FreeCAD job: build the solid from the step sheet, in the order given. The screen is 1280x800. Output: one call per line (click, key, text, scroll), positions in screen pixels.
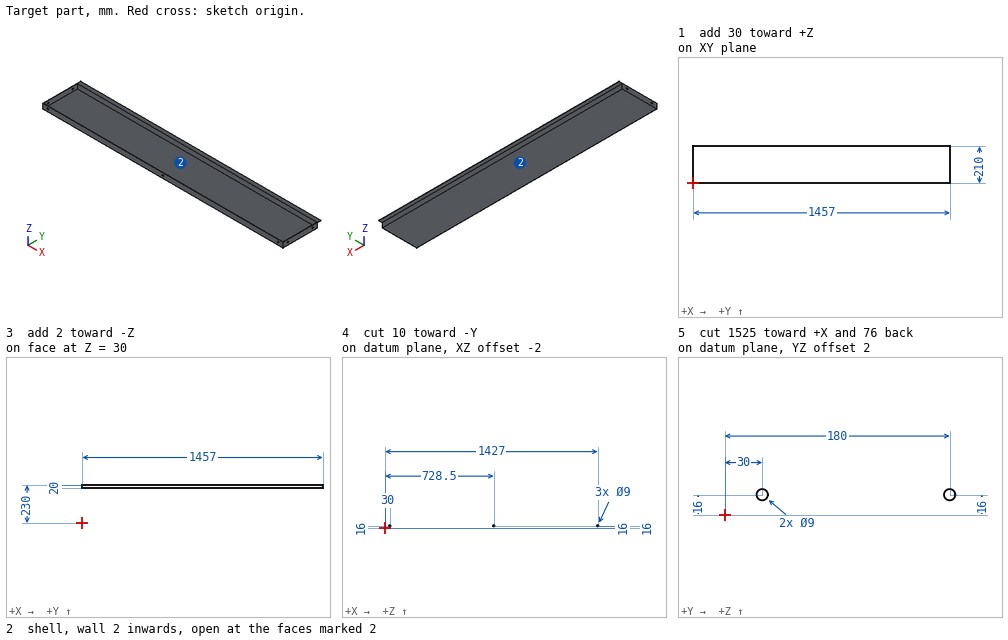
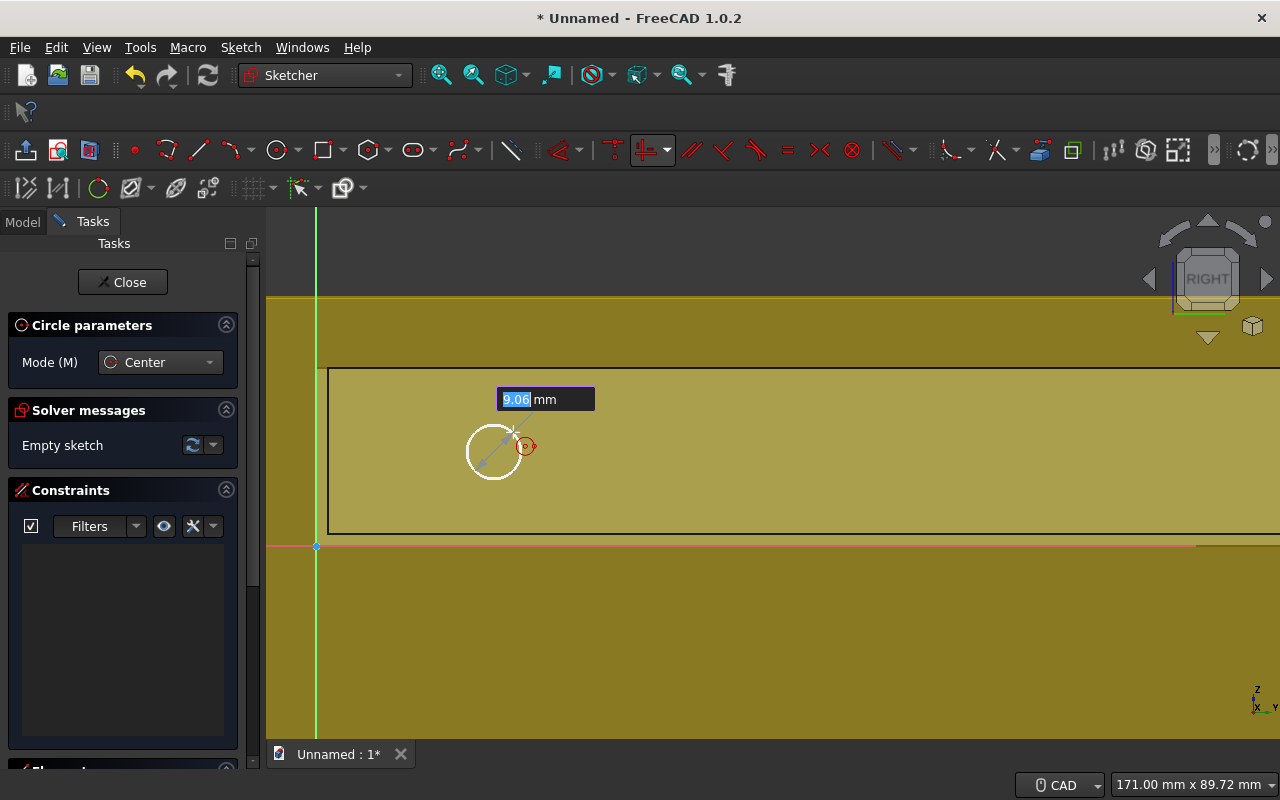
text(9)
key(Return)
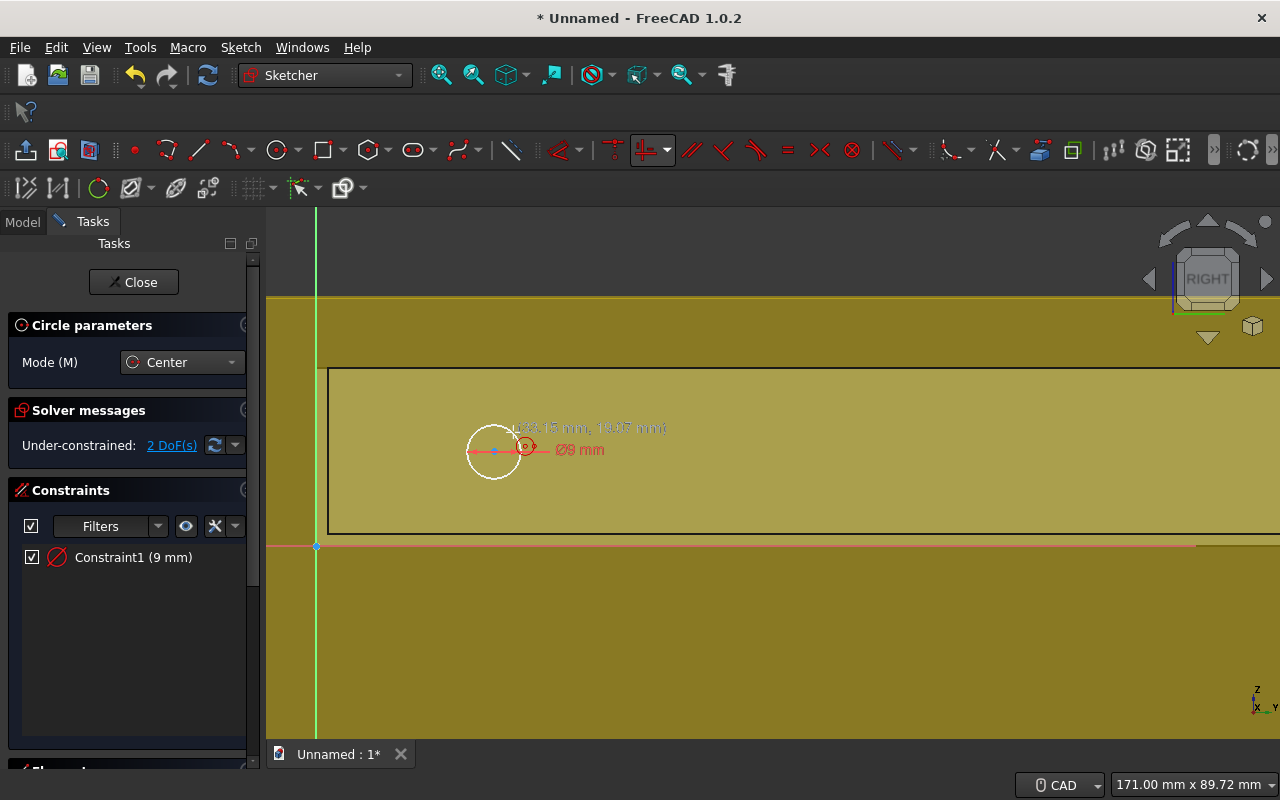
scroll(511, 458, down, 3)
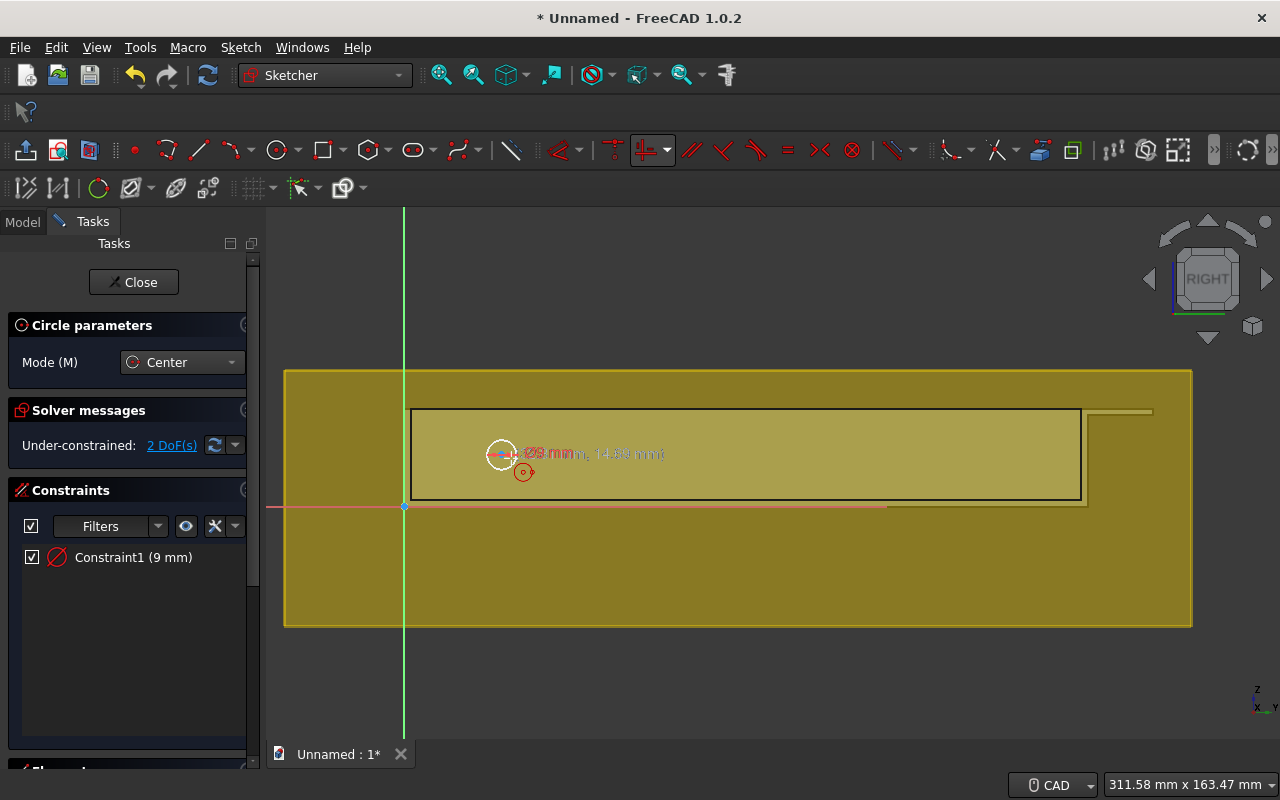
scroll(990, 454, up, 3)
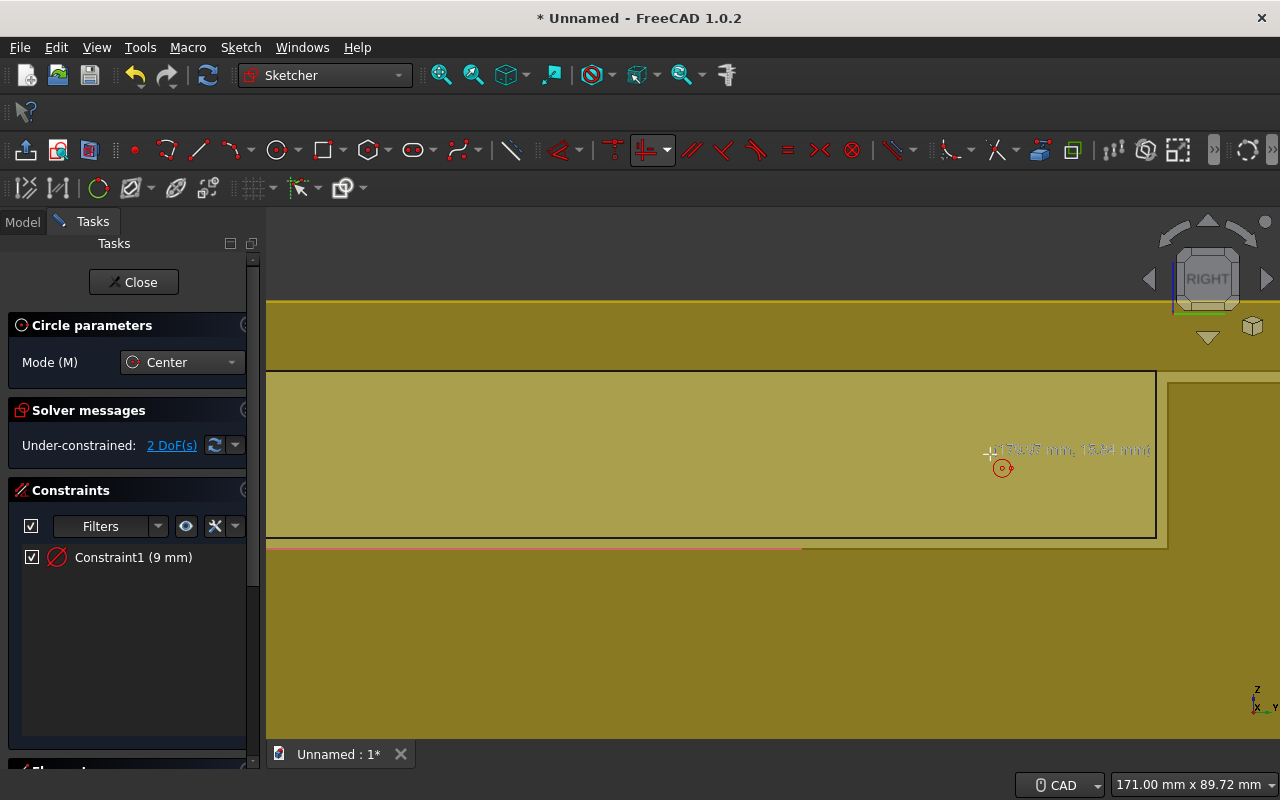
click(990, 455)
move(1008, 436)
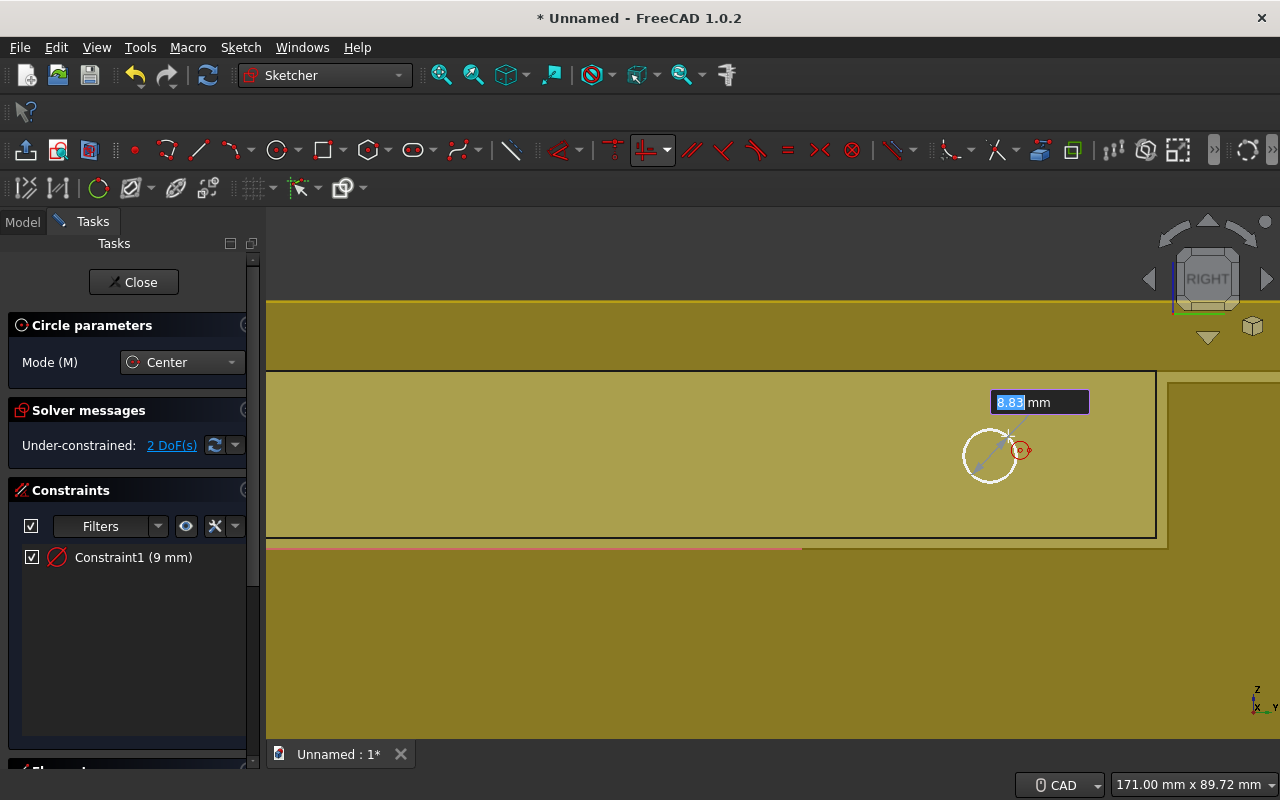
text(9)
key(Return)
key(Escape)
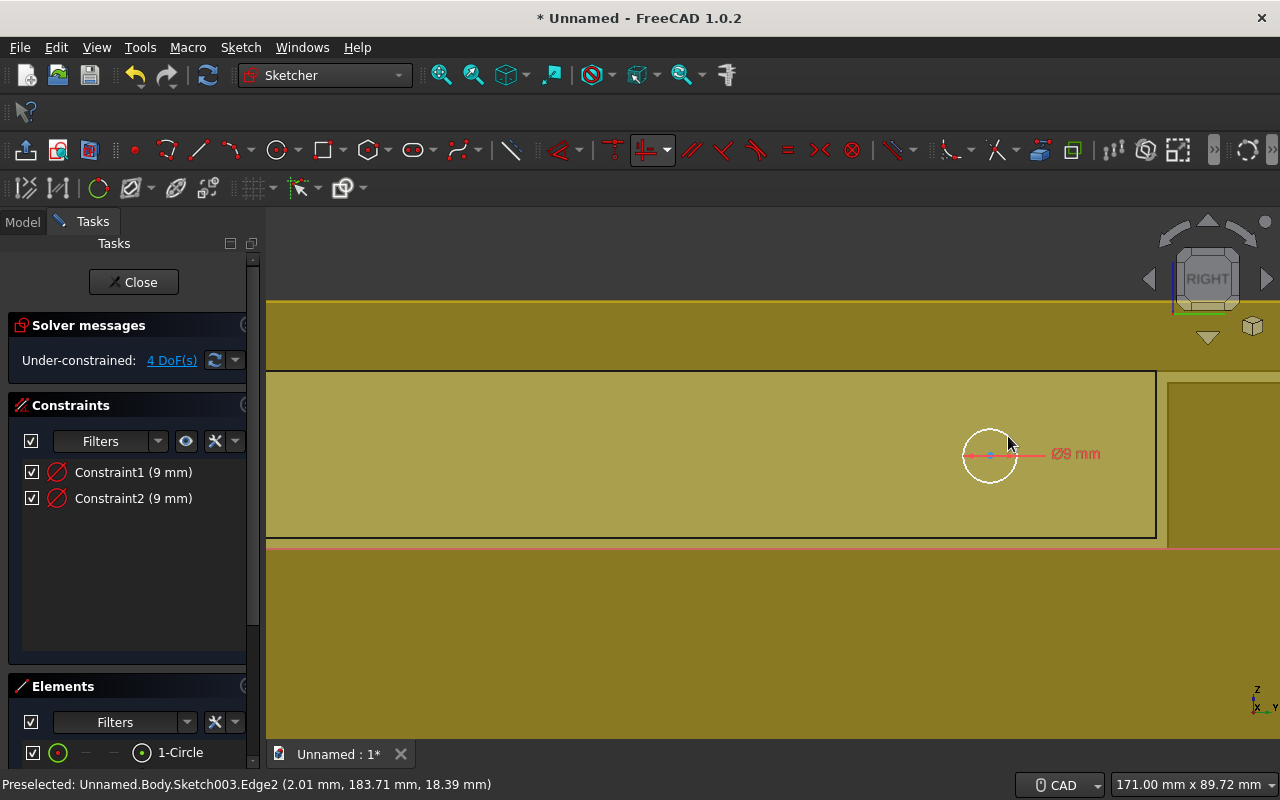
click(558, 150)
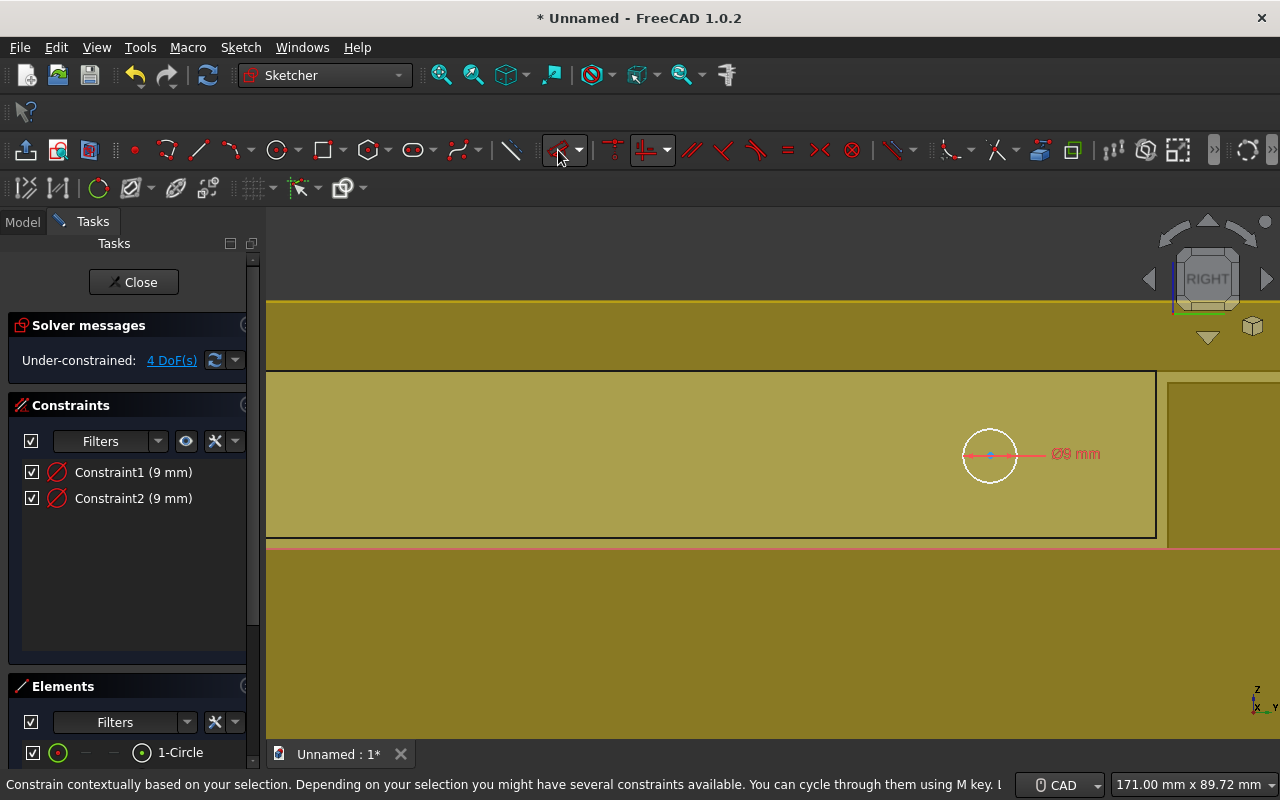
scroll(991, 454, down, 3)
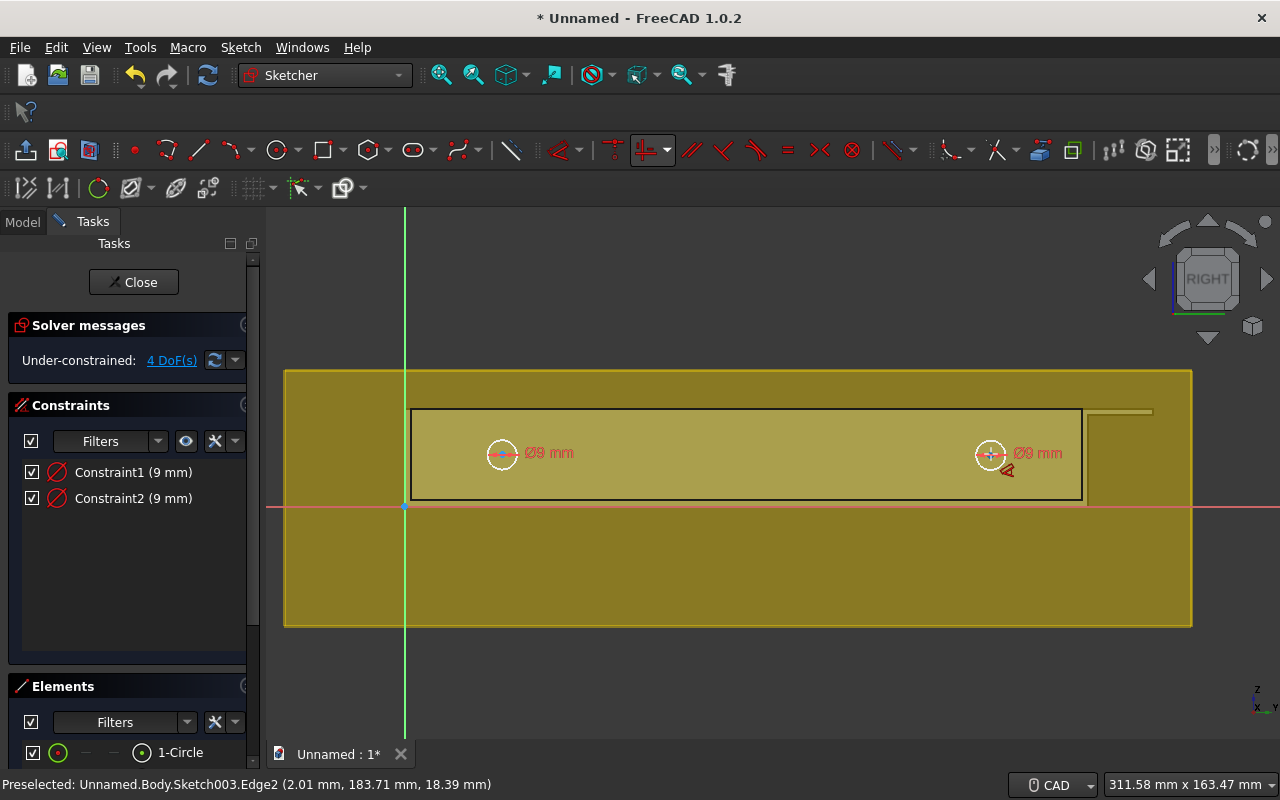
click(502, 455)
click(454, 541)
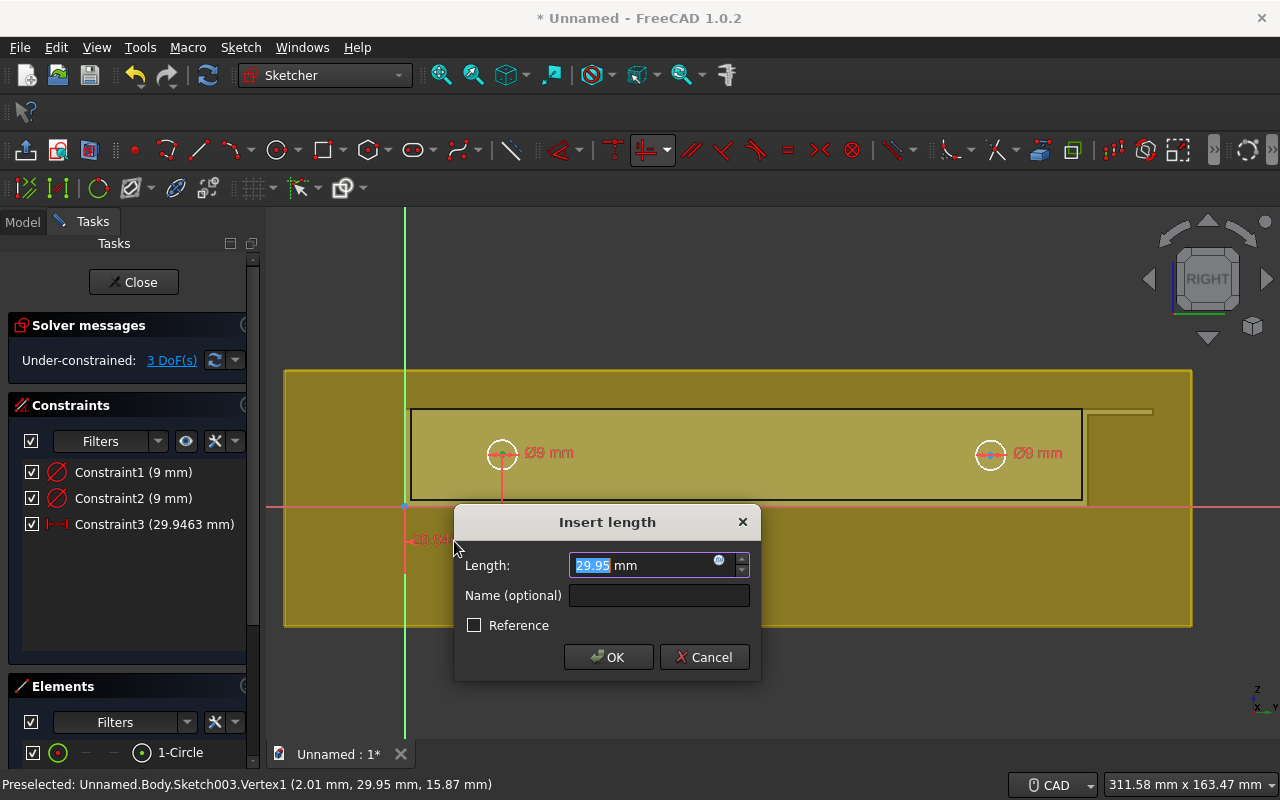
text(30)
key(Return)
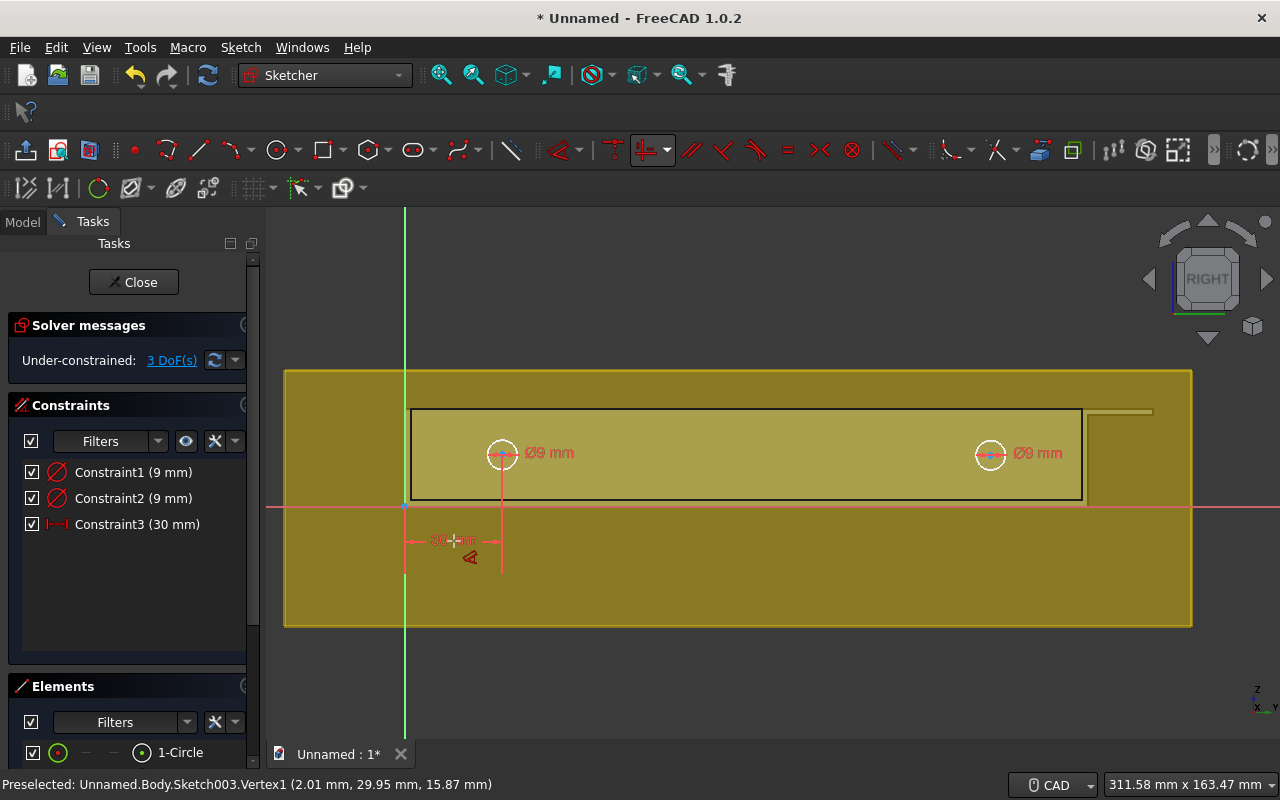
click(502, 455)
click(371, 481)